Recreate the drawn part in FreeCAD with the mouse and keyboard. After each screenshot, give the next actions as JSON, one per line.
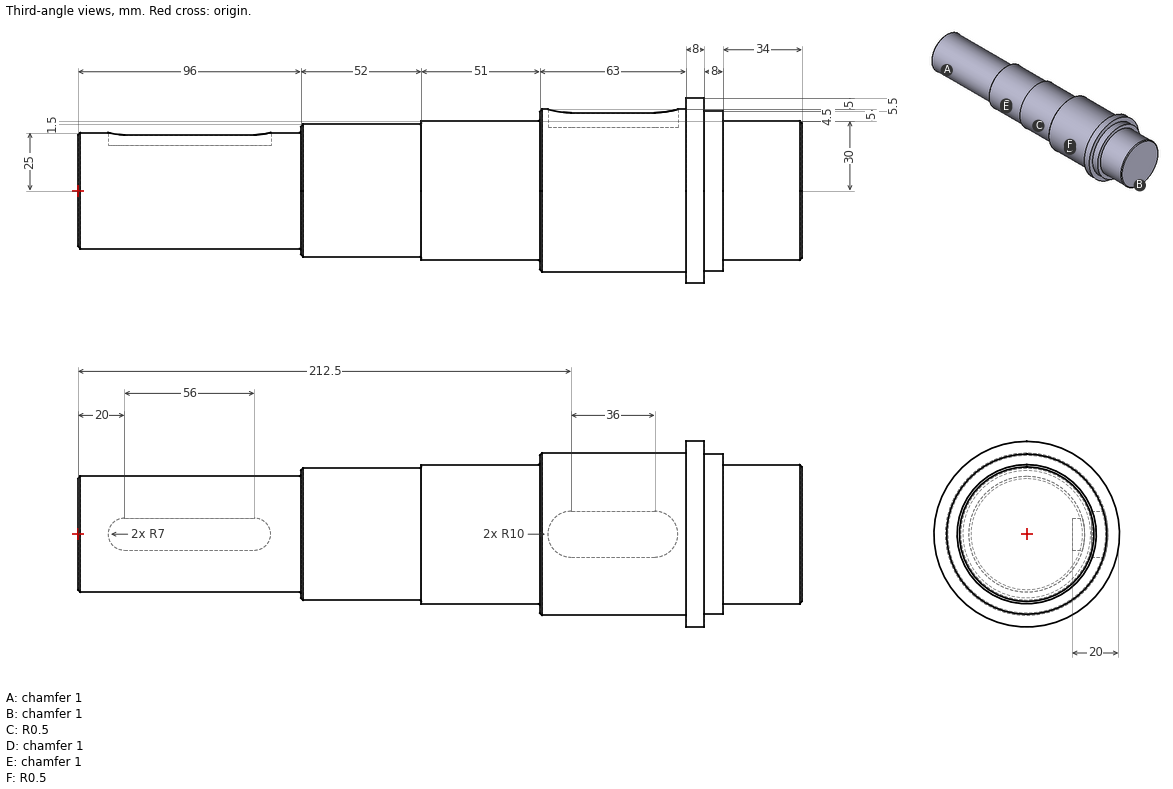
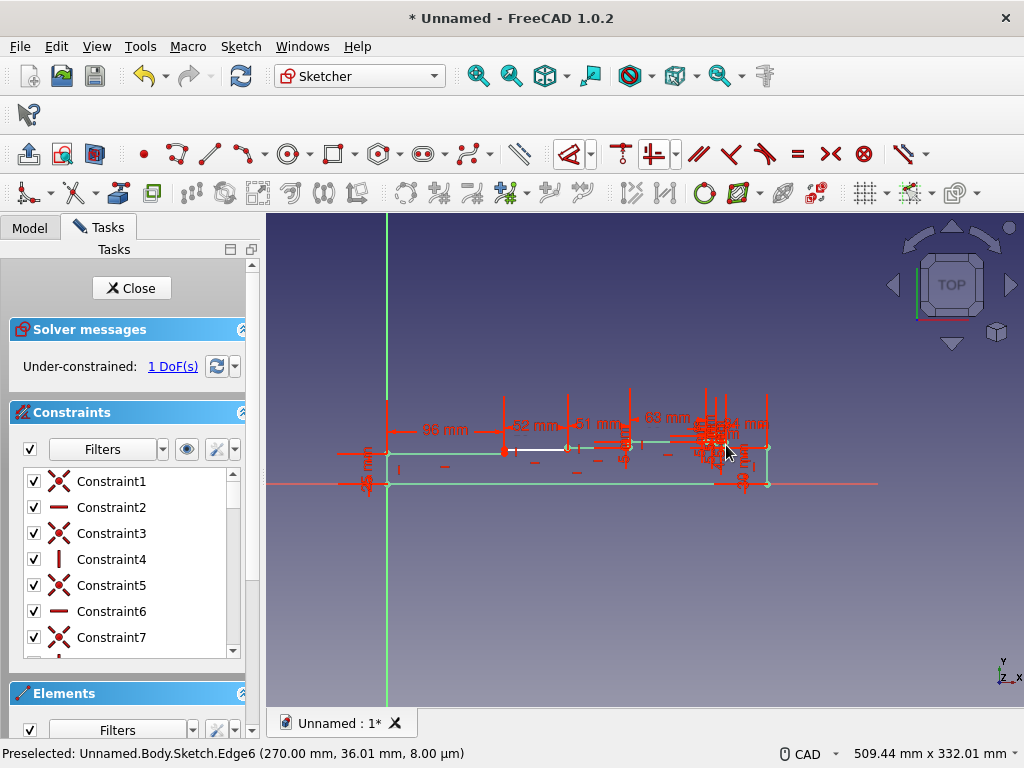
{"action": "scroll", "coordinate": [568, 449], "scroll_direction": "up", "scroll_amount": 16}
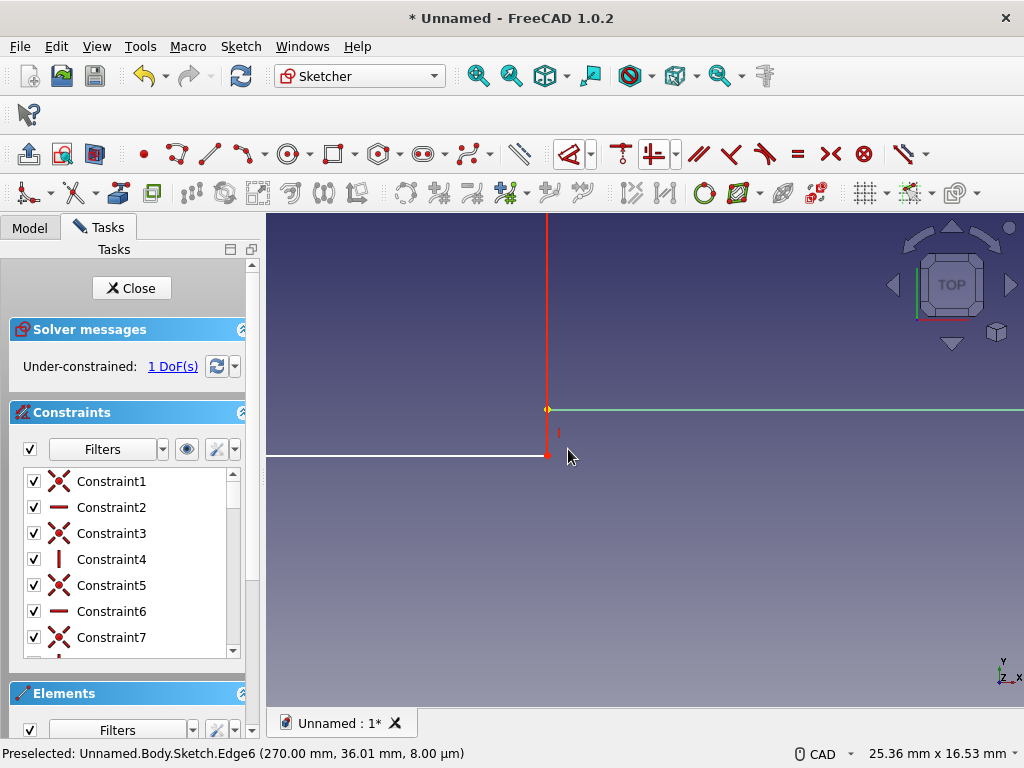
{"action": "left_click", "coordinate": [547, 433]}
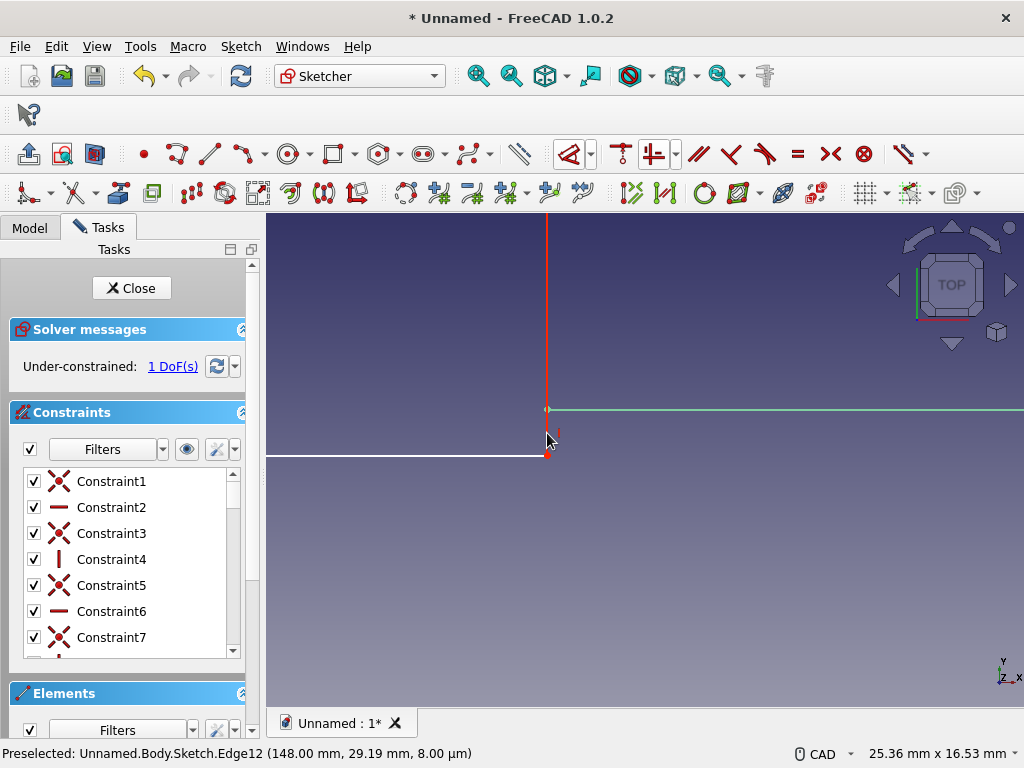
{"action": "key", "text": "i"}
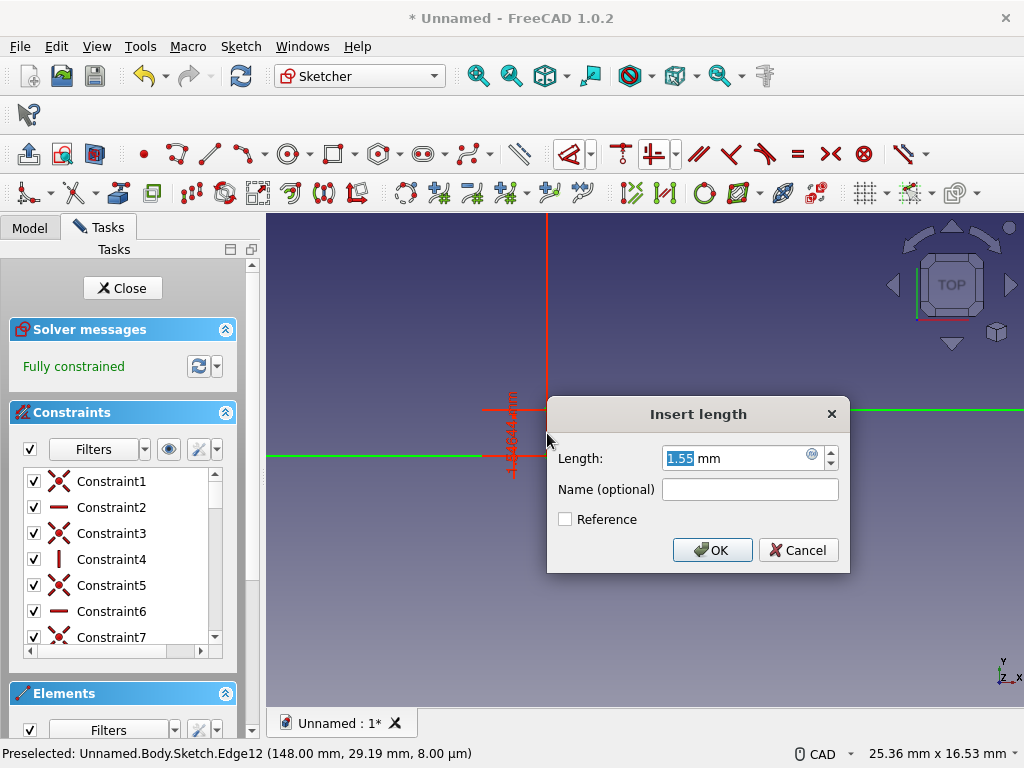
{"action": "type", "text": "1.5"}
{"action": "key", "text": "Return"}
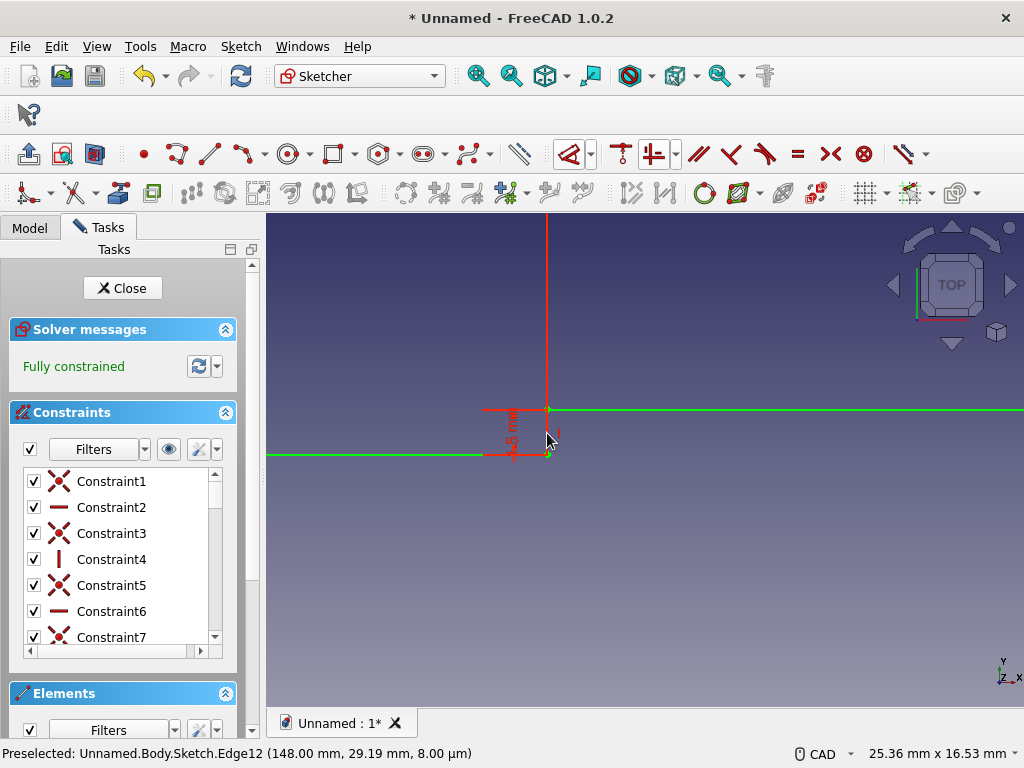
{"action": "left_click", "coordinate": [123, 288]}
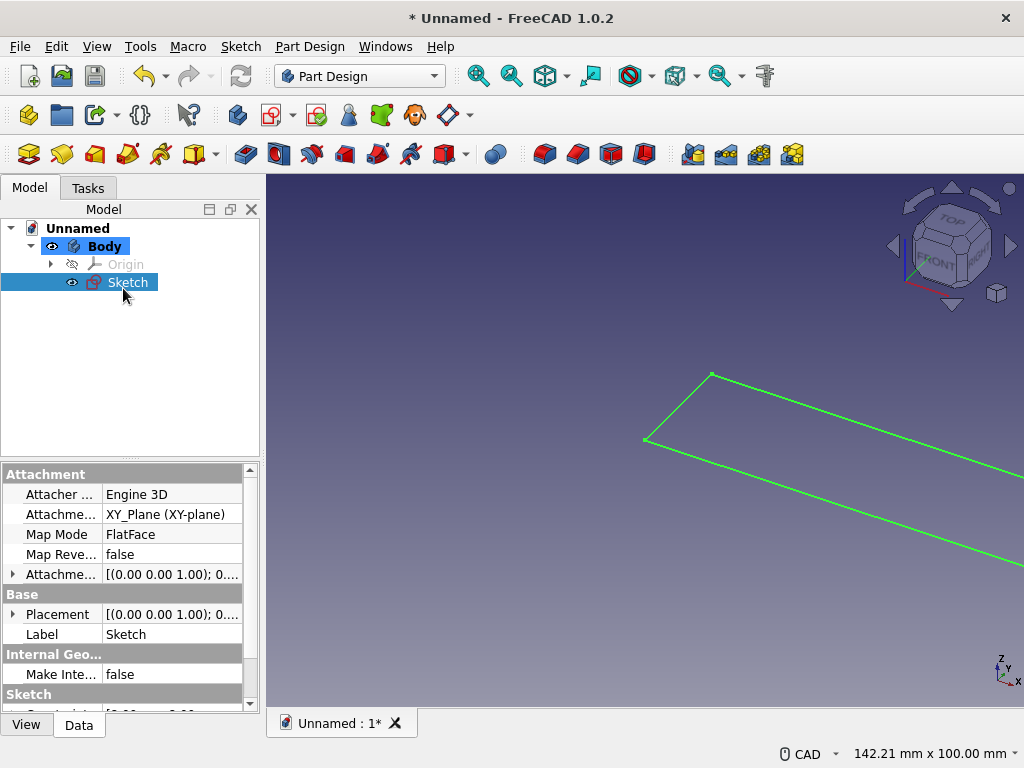
{"action": "left_click", "coordinate": [62, 154]}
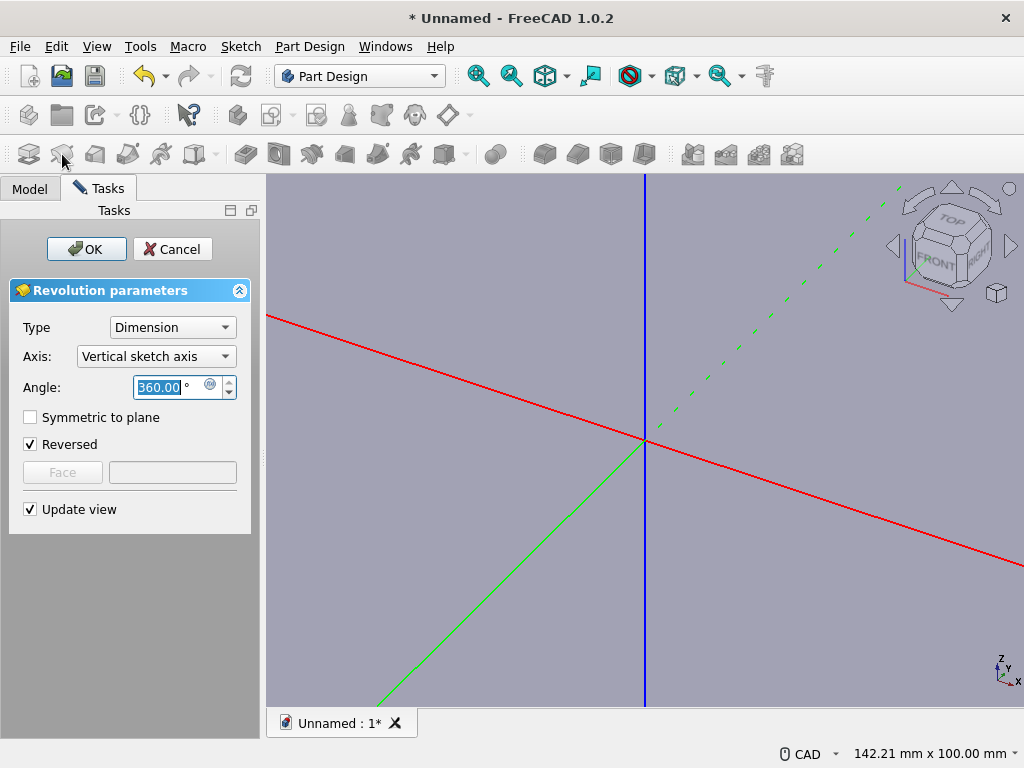
{"action": "left_click", "coordinate": [157, 356]}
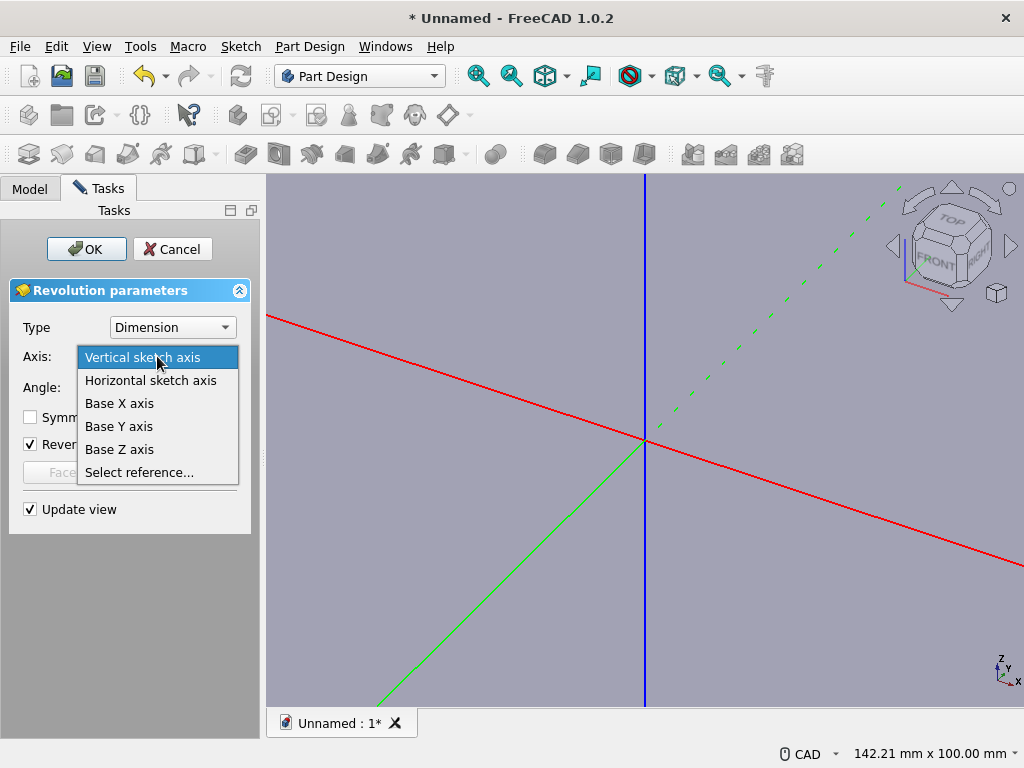
{"action": "left_click", "coordinate": [156, 380]}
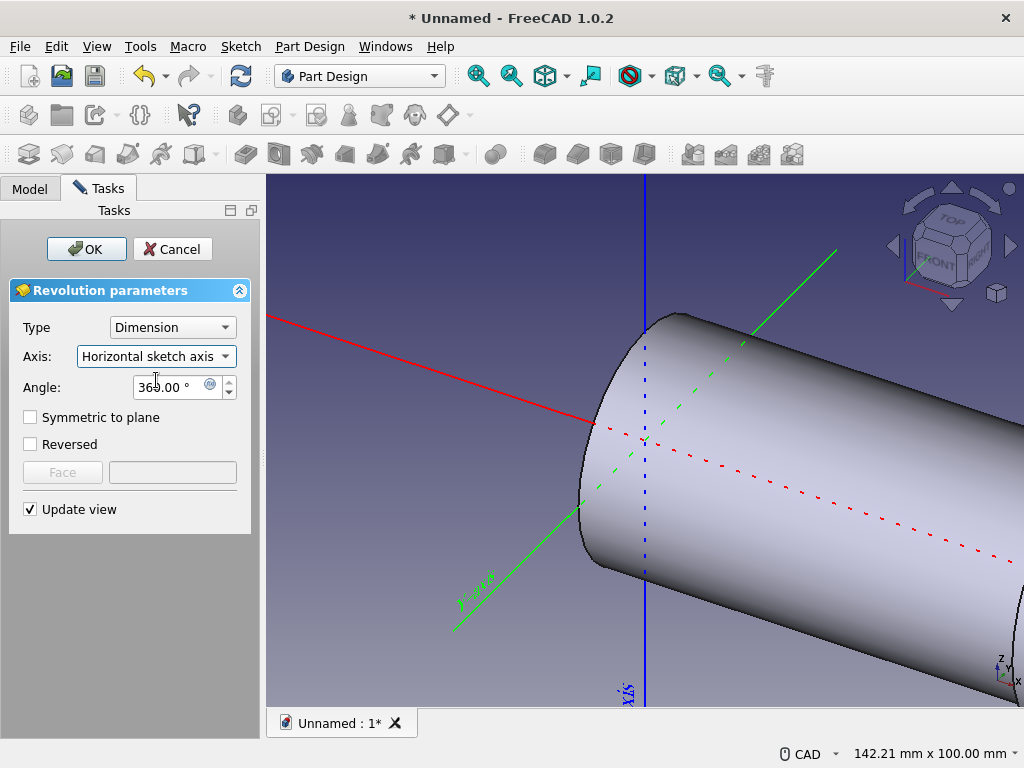
{"action": "left_click", "coordinate": [87, 249]}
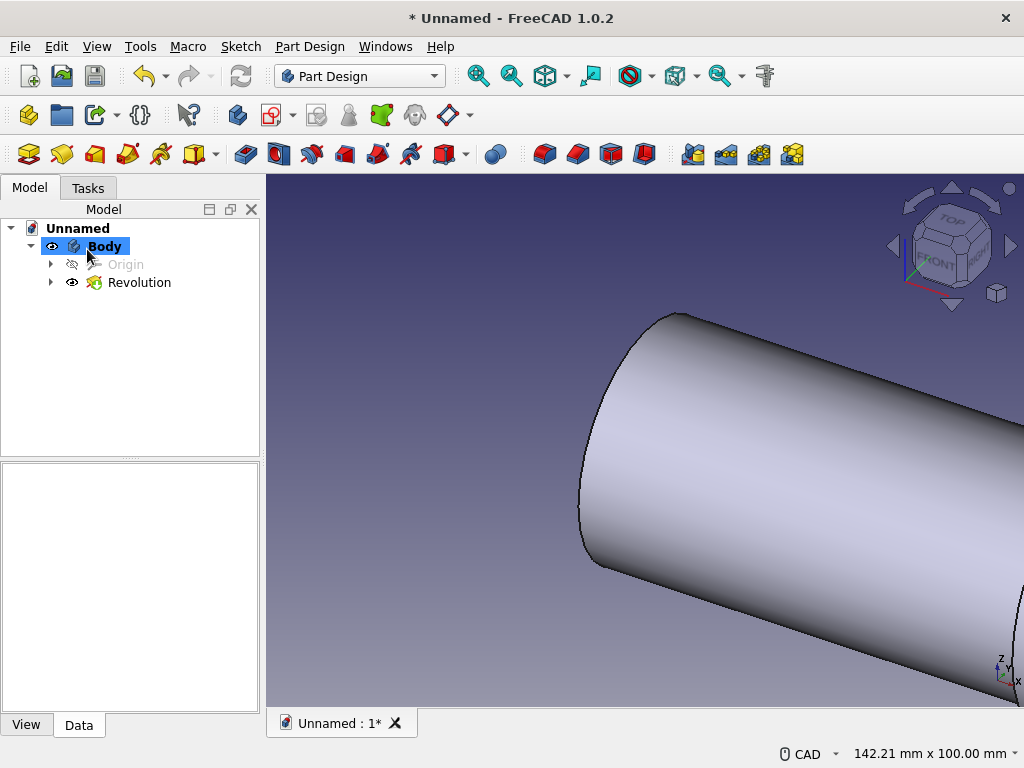
{"action": "left_click", "coordinate": [479, 76]}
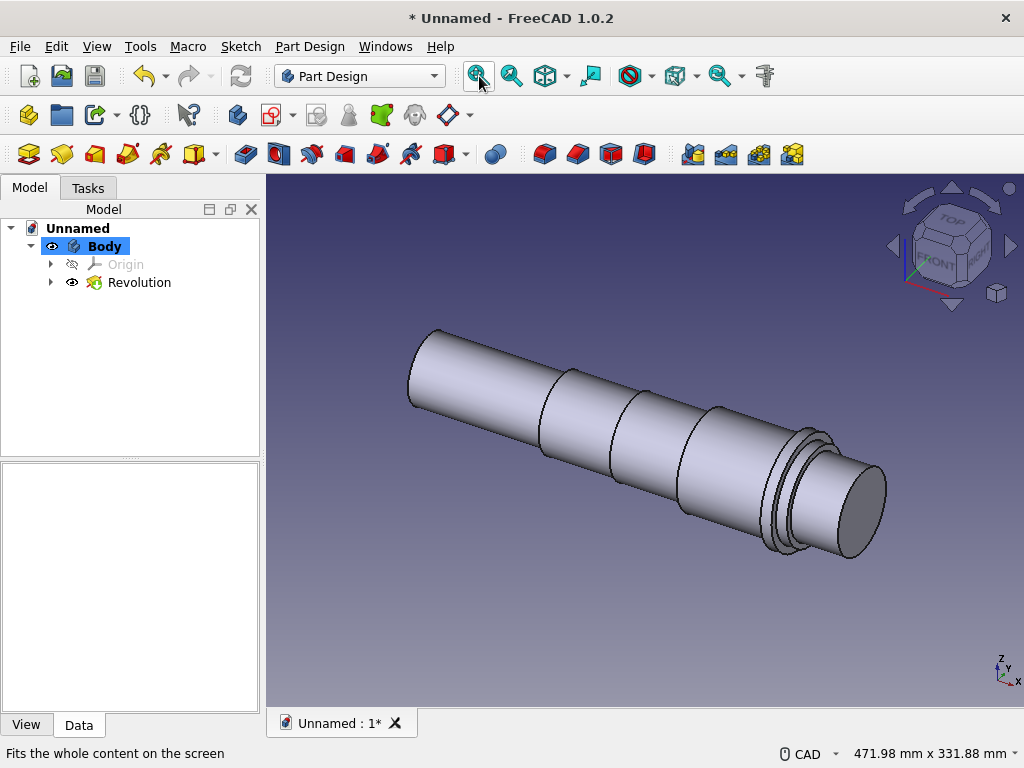
{"action": "left_click", "coordinate": [434, 330]}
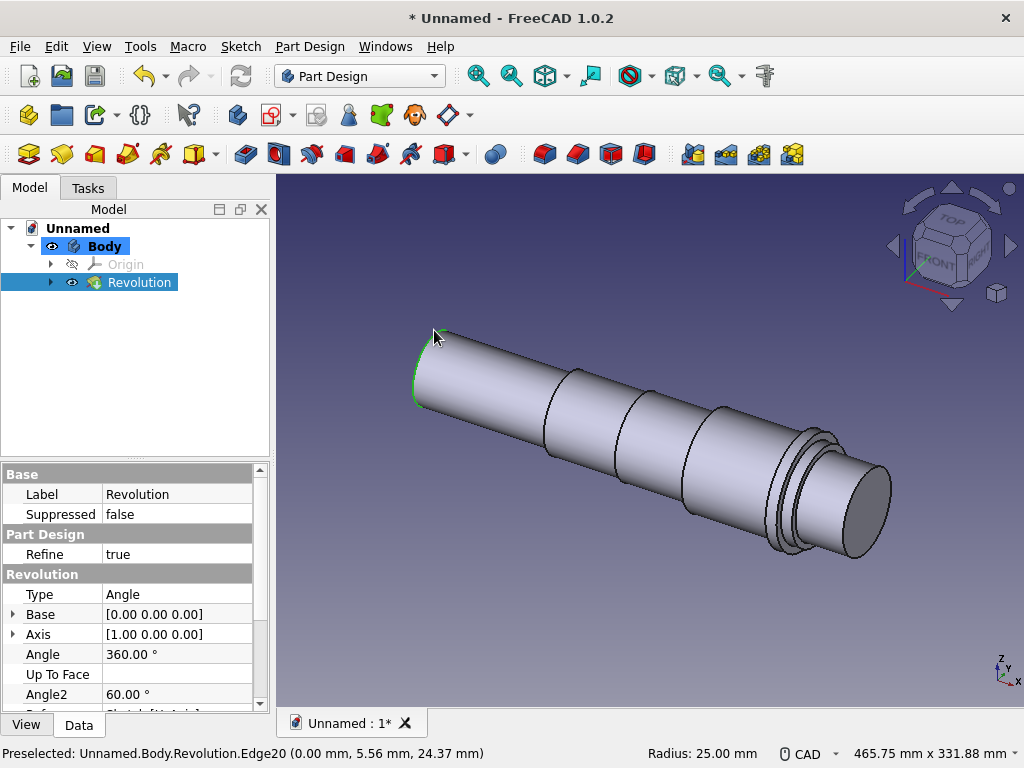
{"action": "left_click", "coordinate": [578, 154]}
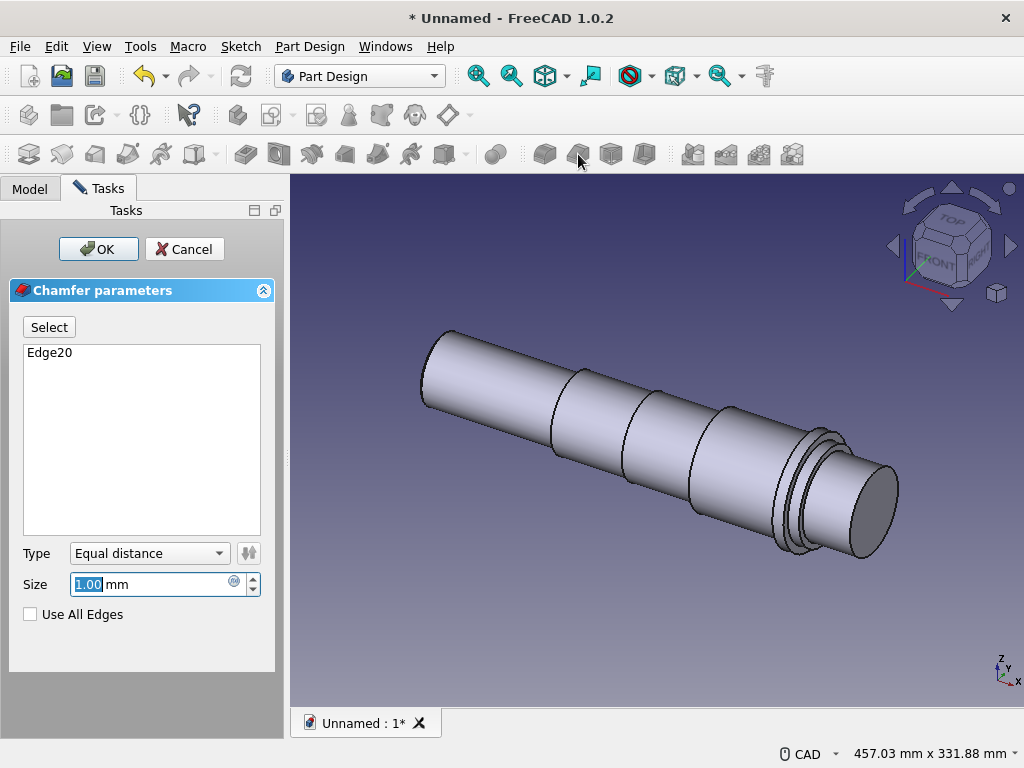
{"action": "type", "text": "1"}
{"action": "key", "text": "Tab"}